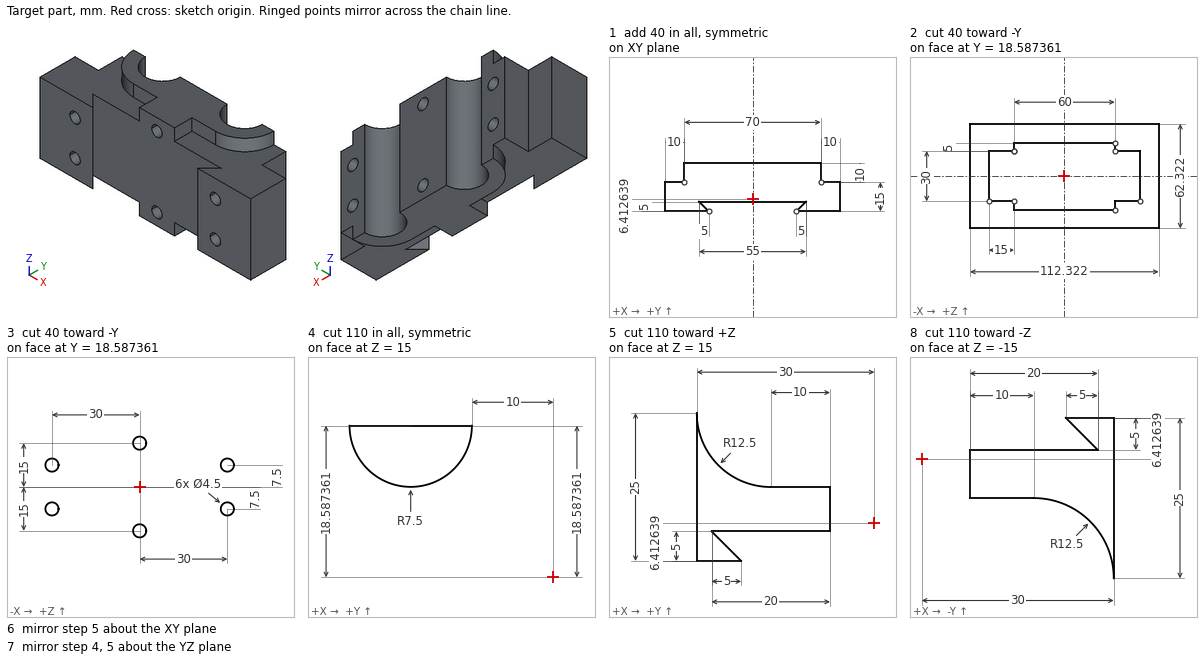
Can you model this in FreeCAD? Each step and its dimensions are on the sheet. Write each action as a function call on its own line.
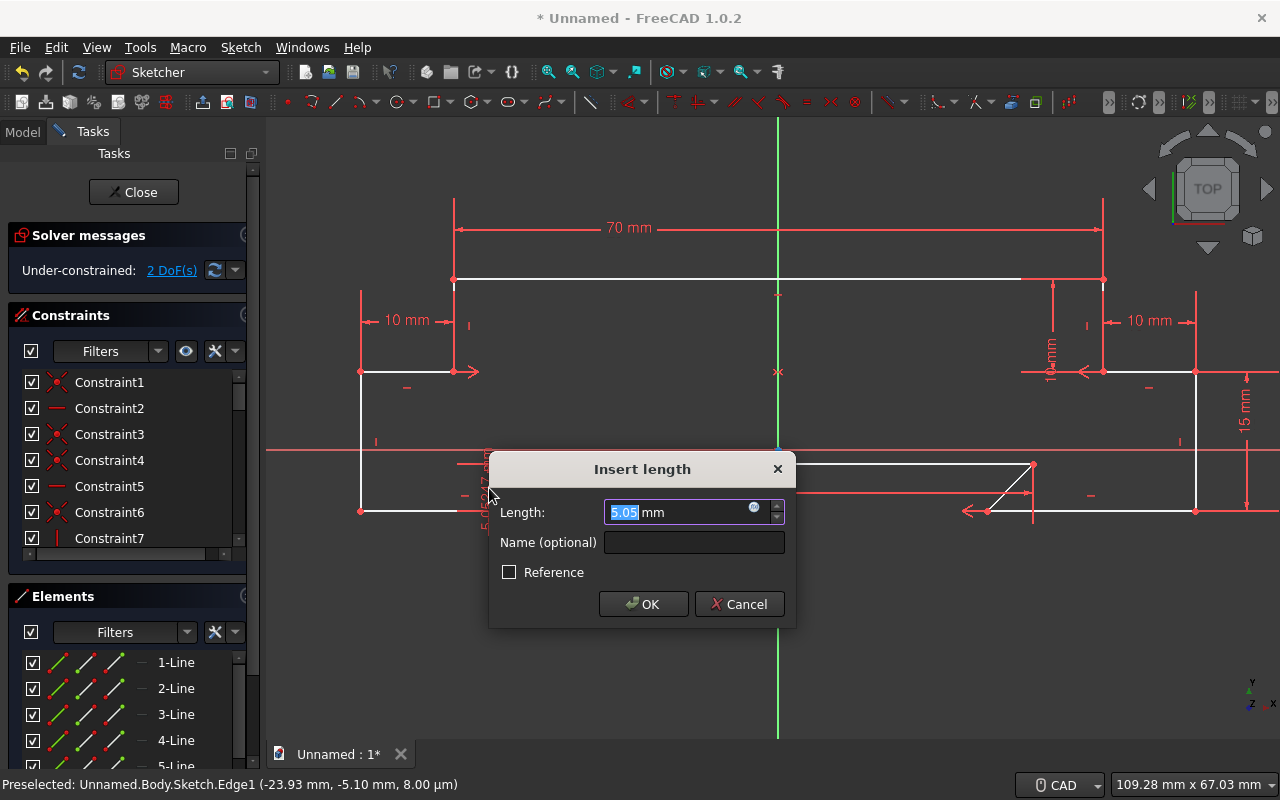
text(5)
key(Return)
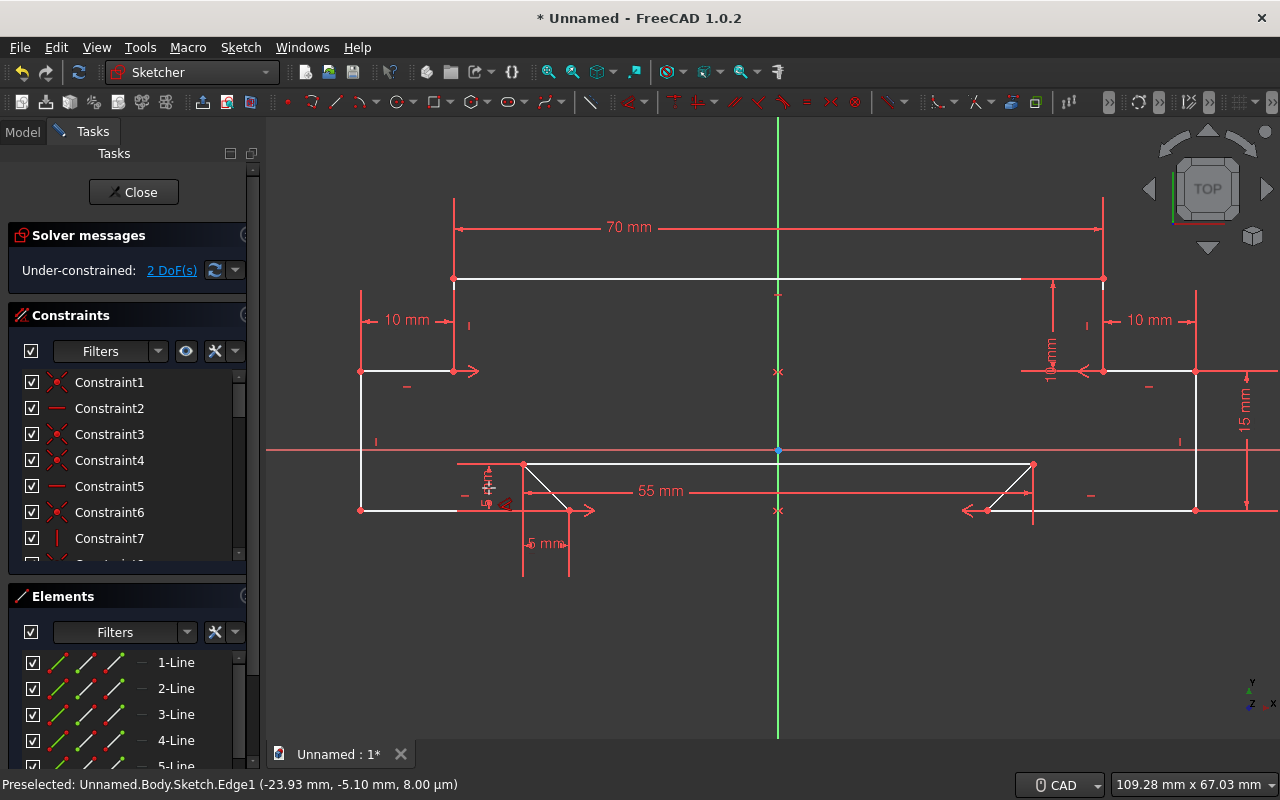
click(1020, 478)
click(1010, 545)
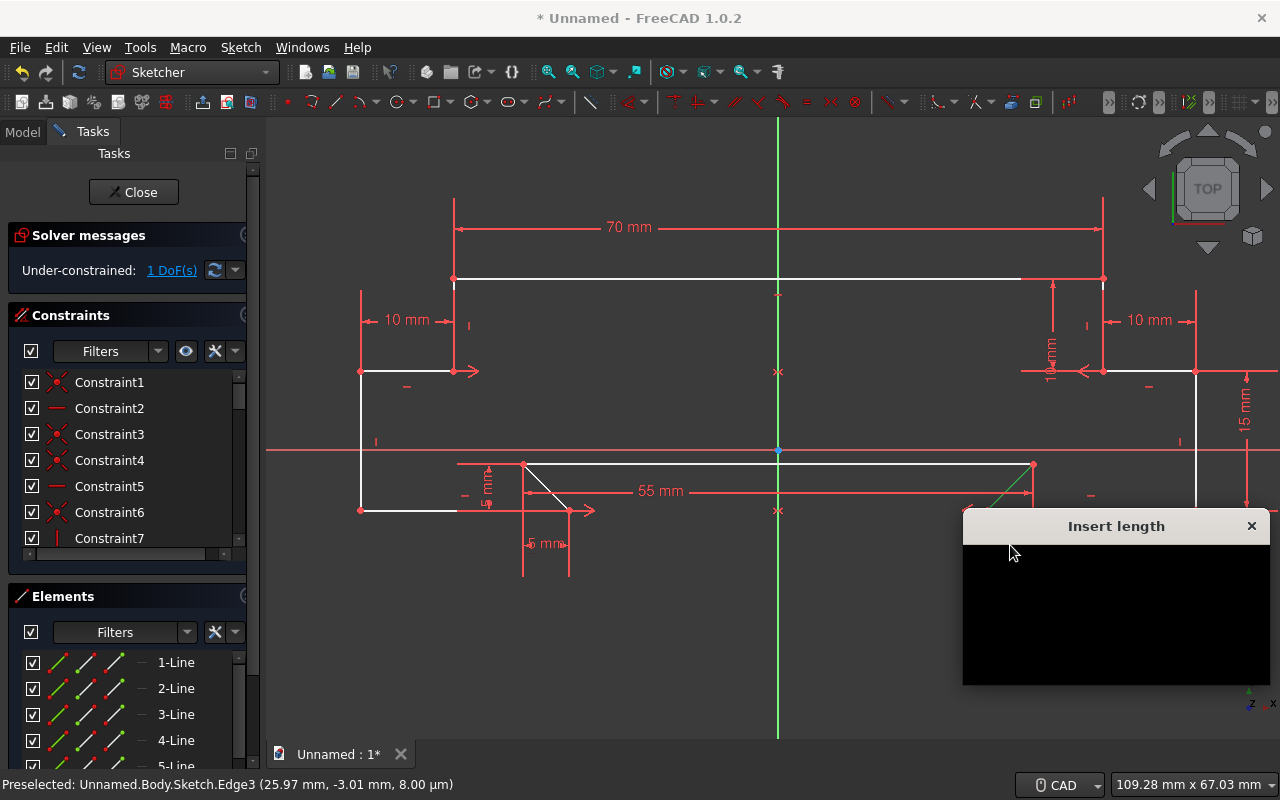
text(5)
key(Return)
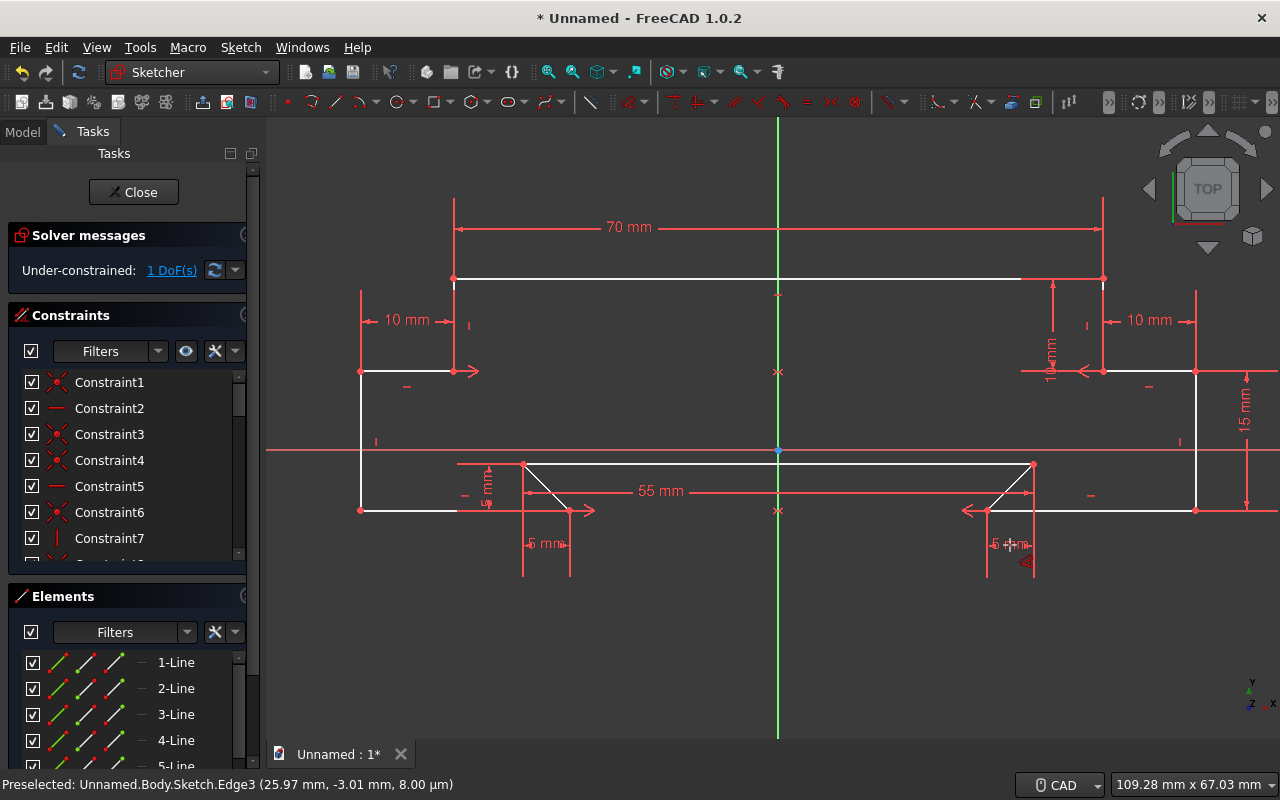
click(570, 511)
click(812, 480)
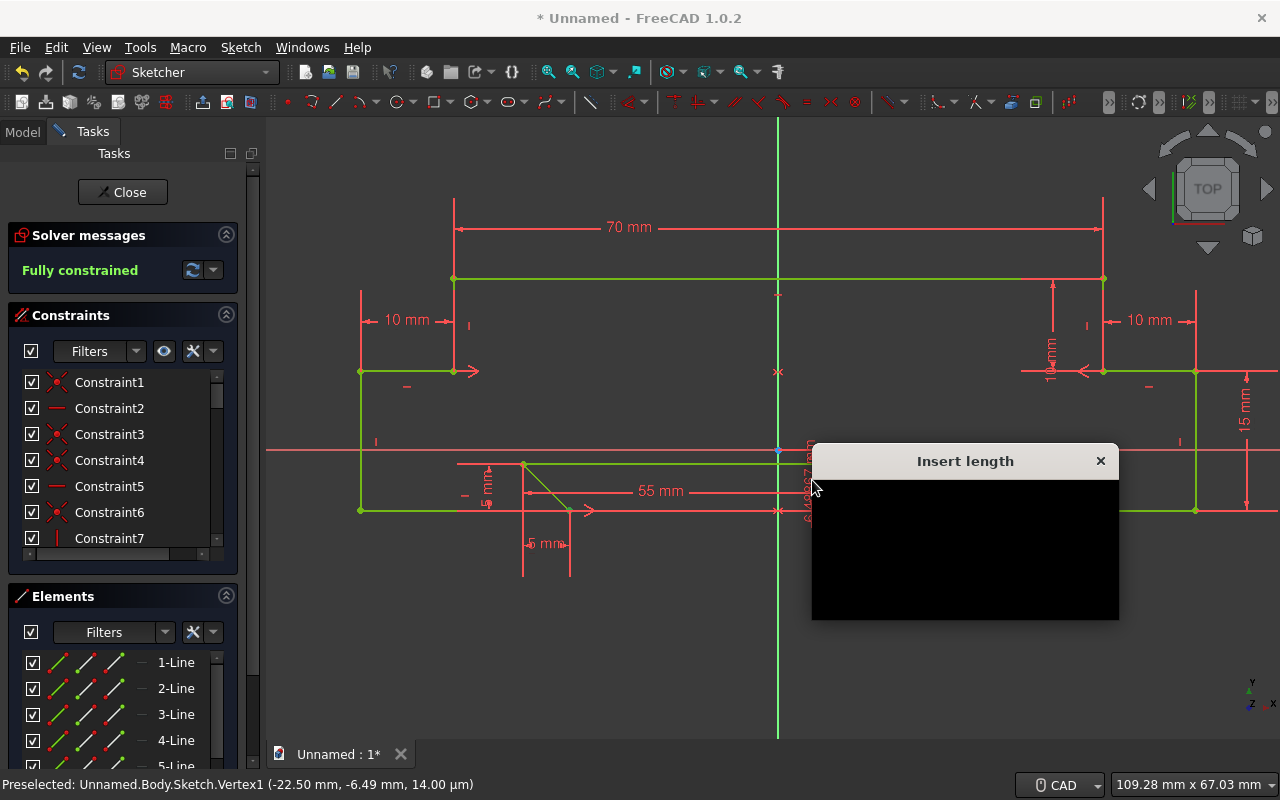
text(6.412639)
key(Return)
key(Escape)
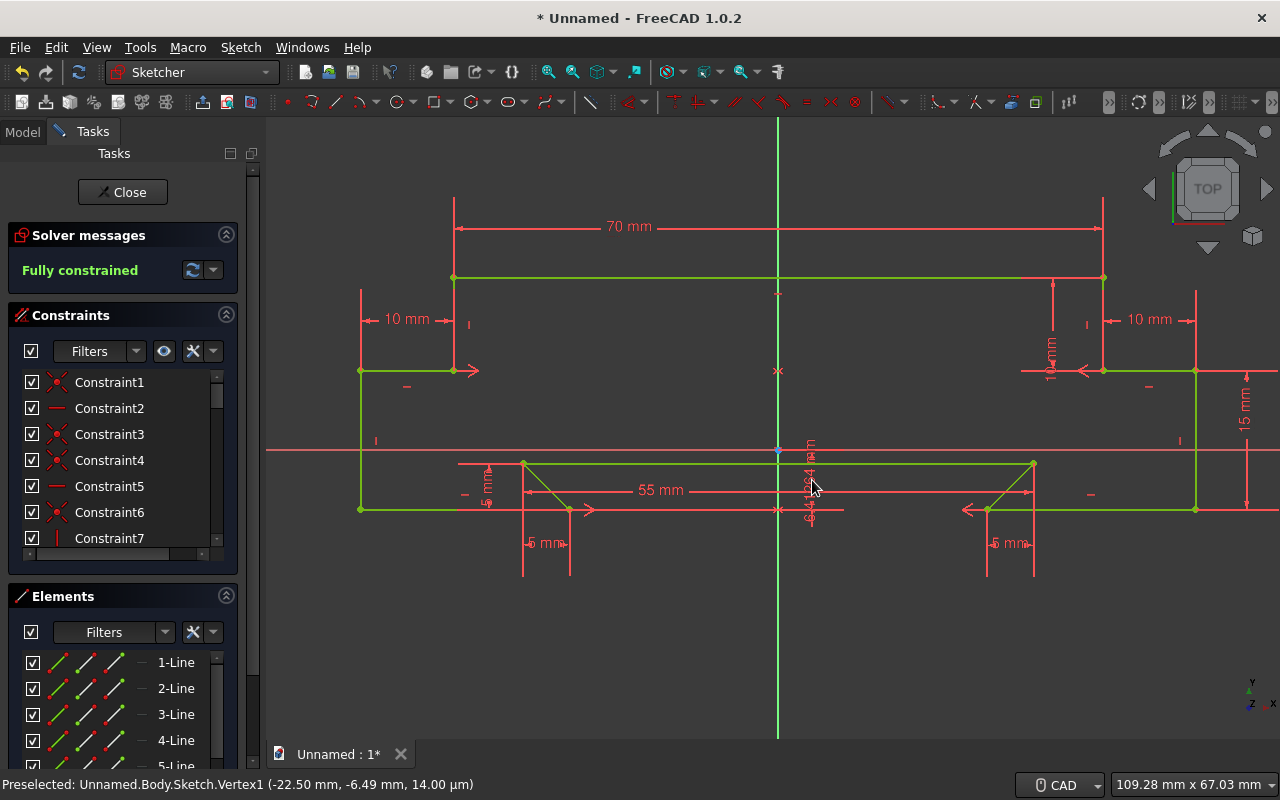
click(123, 192)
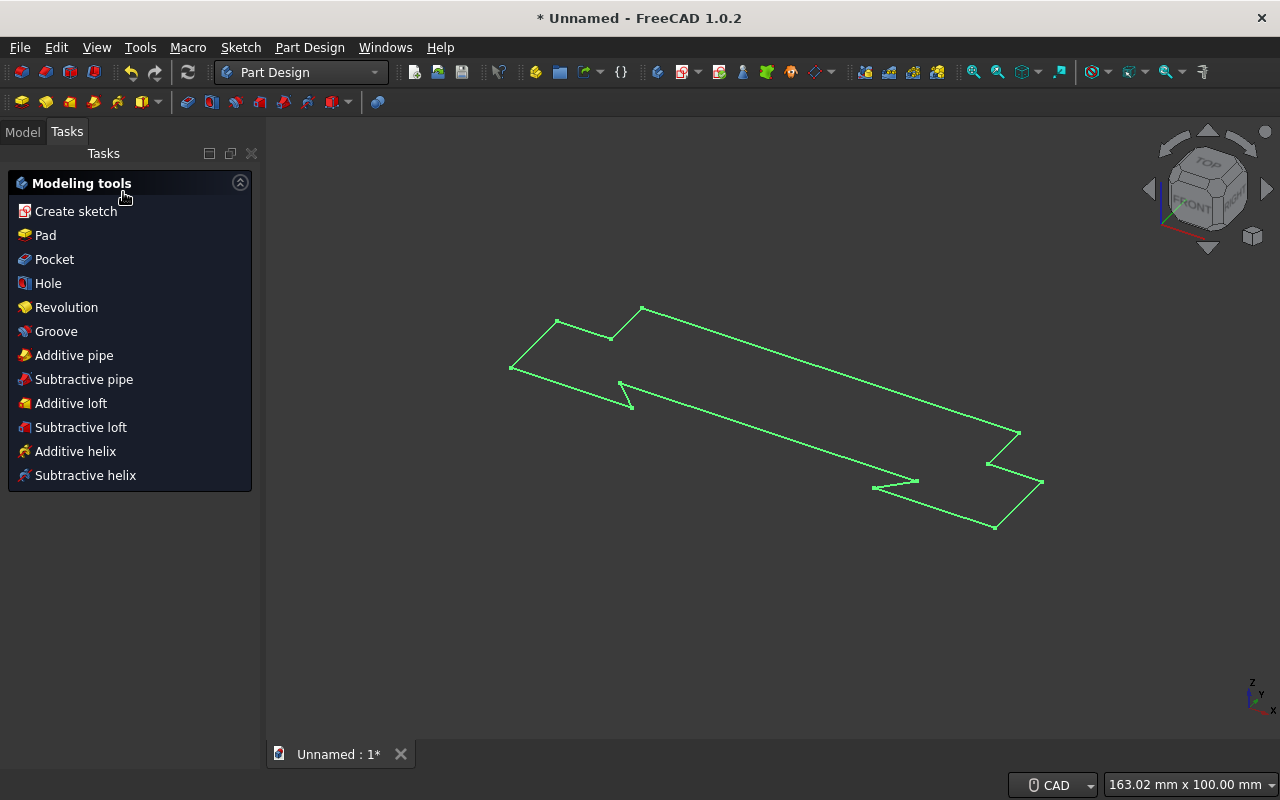
click(22, 102)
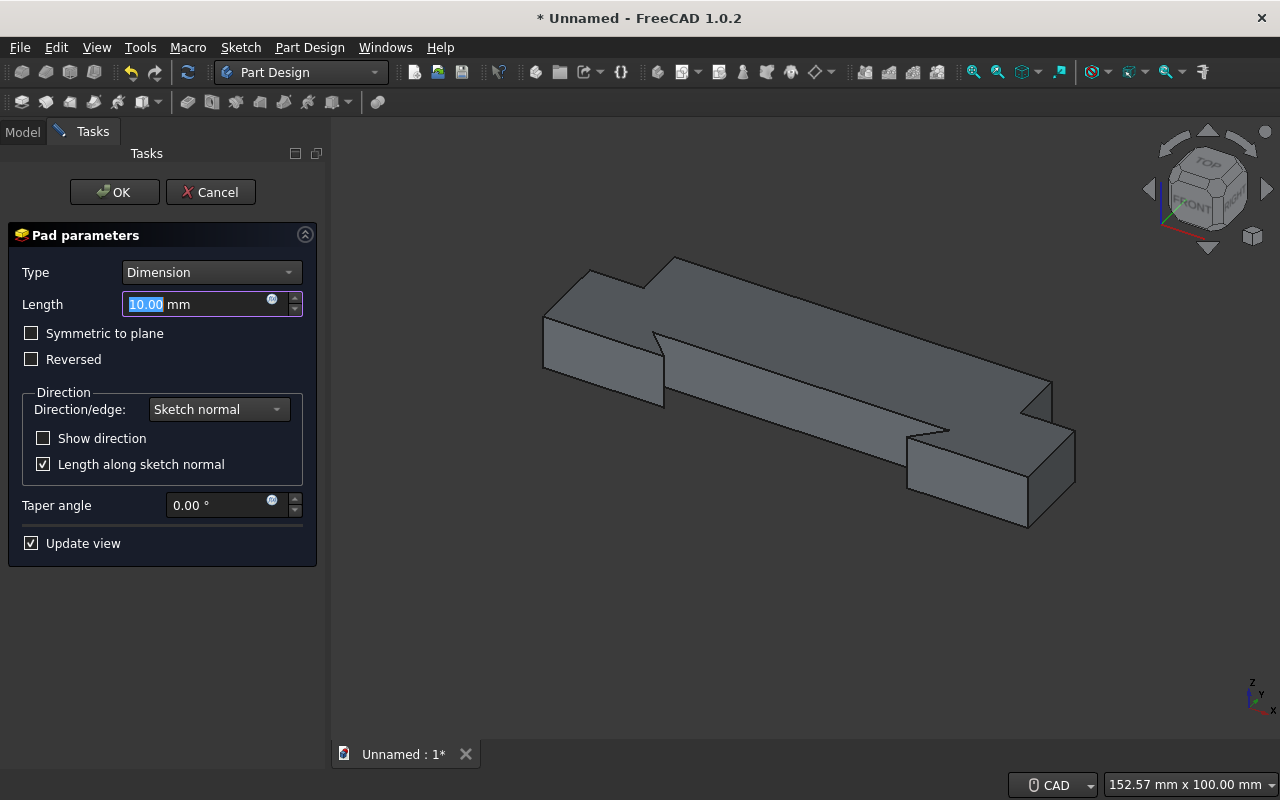
text(40)
key(Tab)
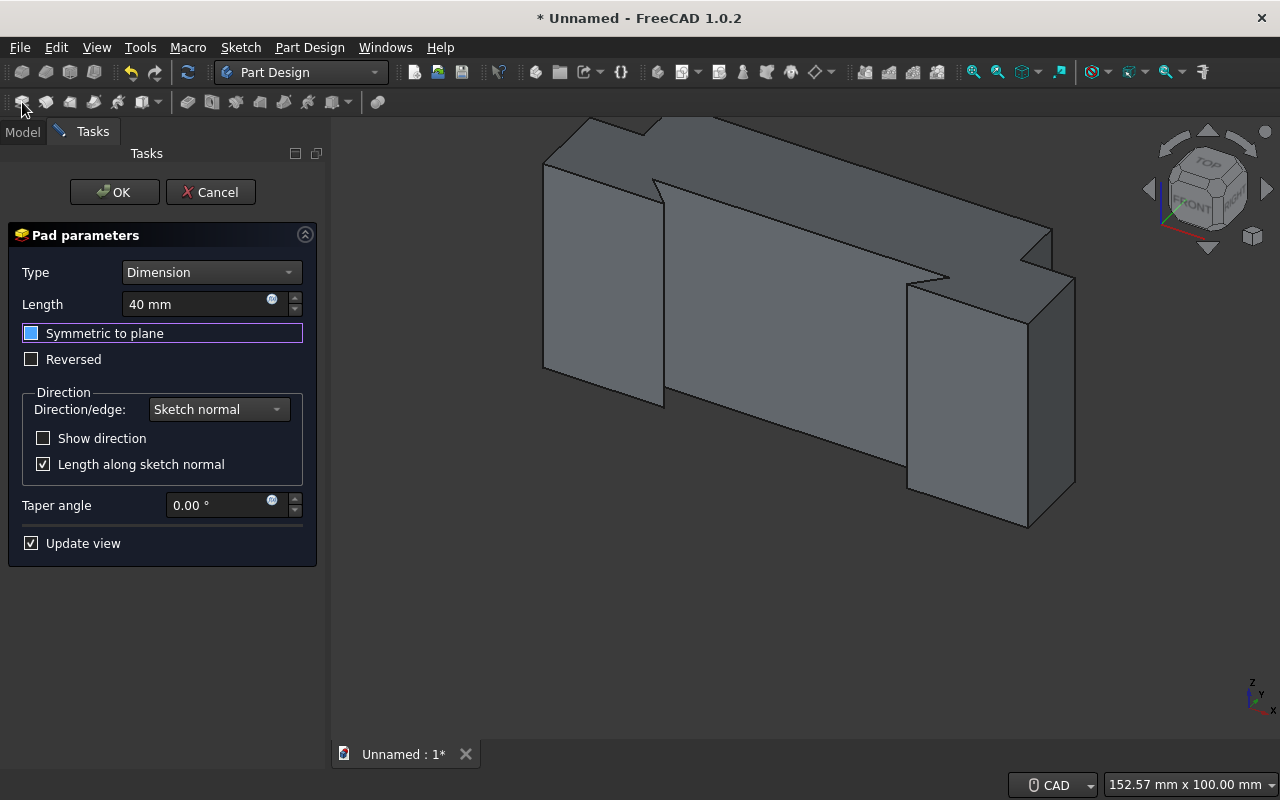
click(30, 333)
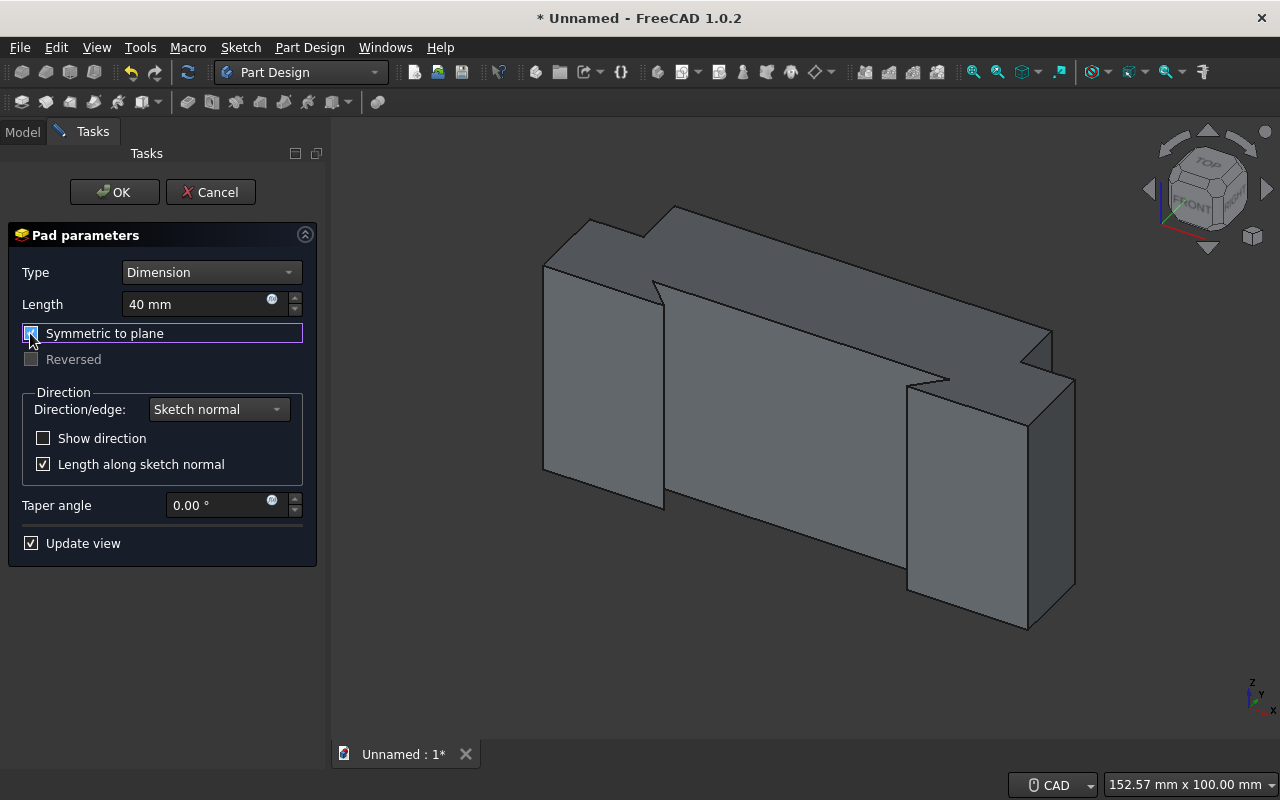
click(115, 192)